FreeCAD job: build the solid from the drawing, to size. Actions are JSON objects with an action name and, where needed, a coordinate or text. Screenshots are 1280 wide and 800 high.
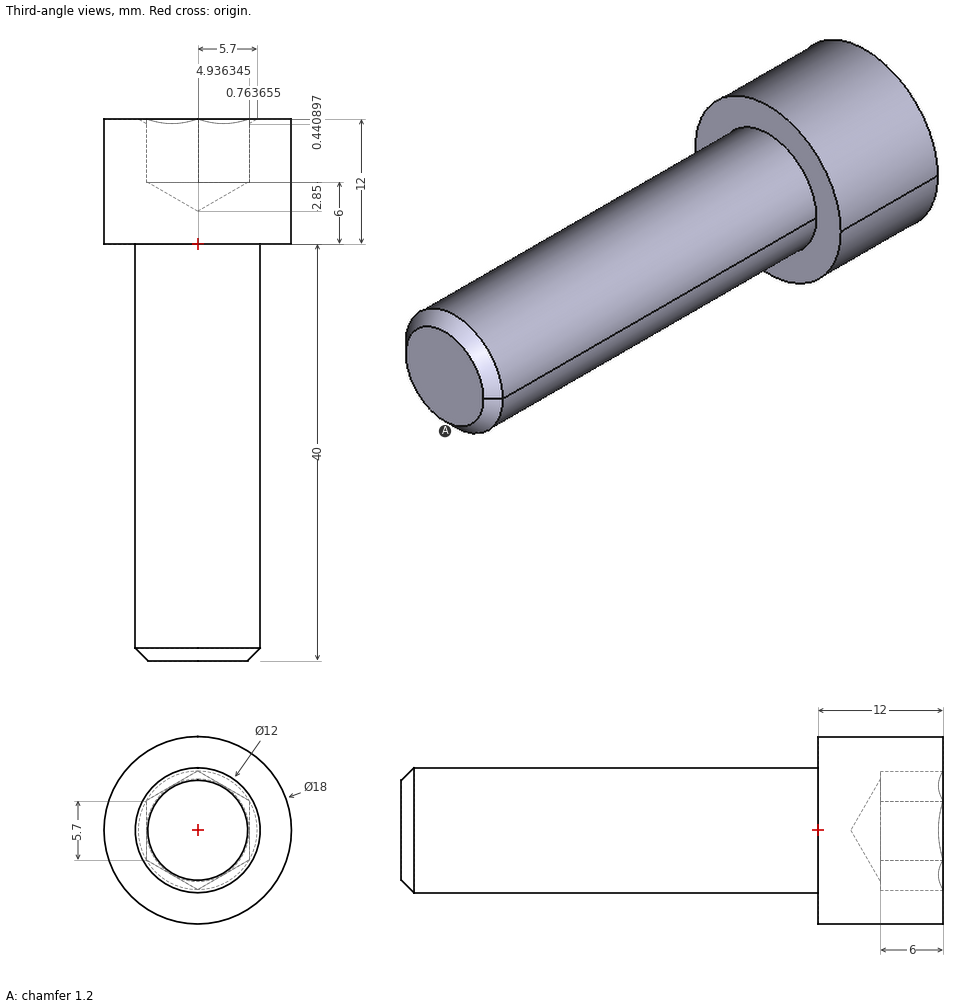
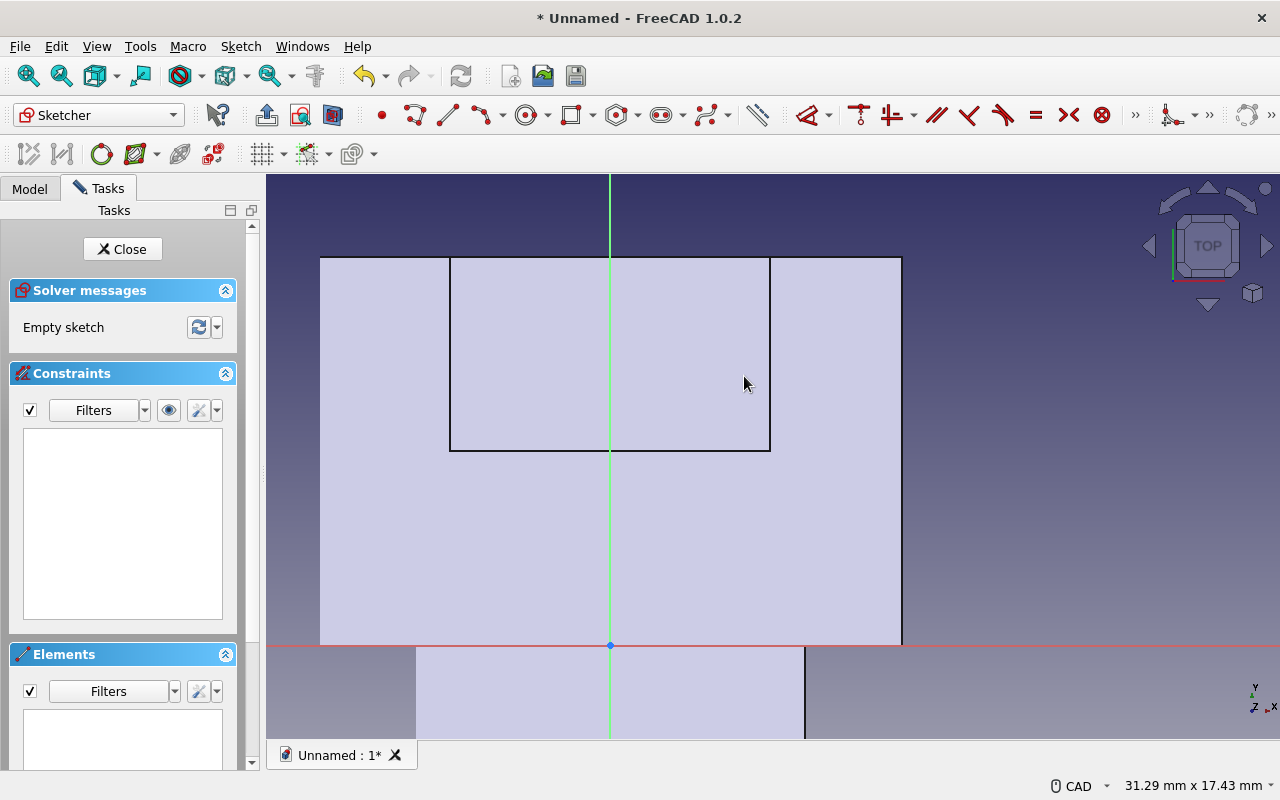
{"action": "left_click", "coordinate": [415, 116]}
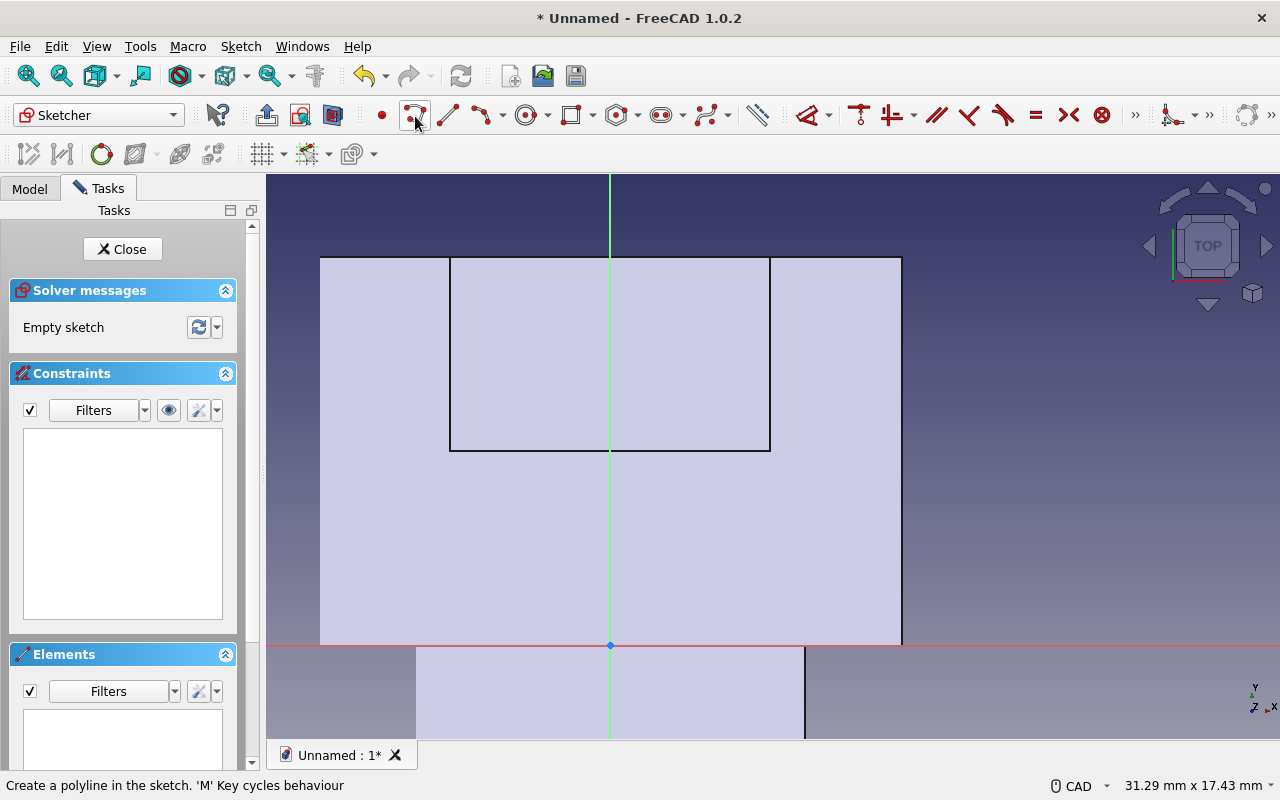
{"action": "left_click", "coordinate": [610, 544]}
{"action": "left_click", "coordinate": [770, 451]}
{"action": "left_click", "coordinate": [619, 451]}
{"action": "left_click", "coordinate": [610, 545]}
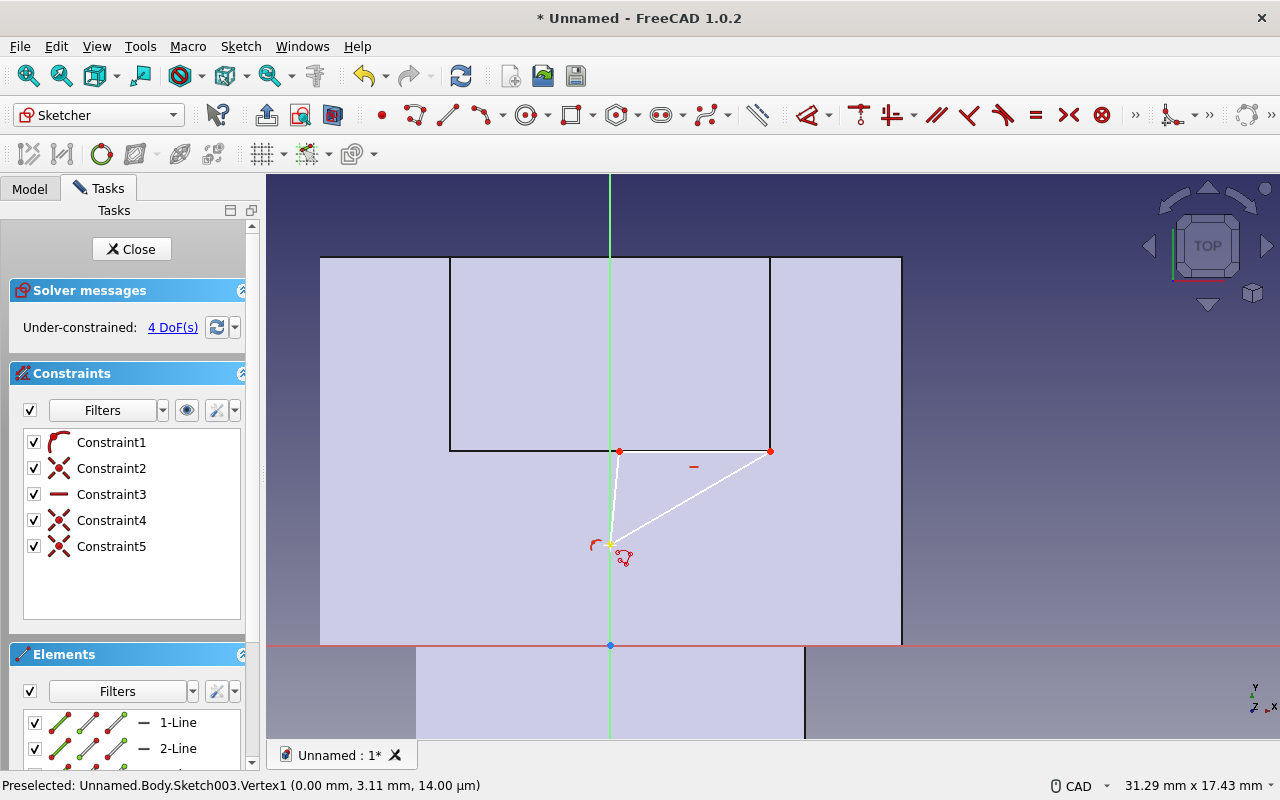
{"action": "left_click", "coordinate": [770, 271]}
{"action": "left_click", "coordinate": [795, 257]}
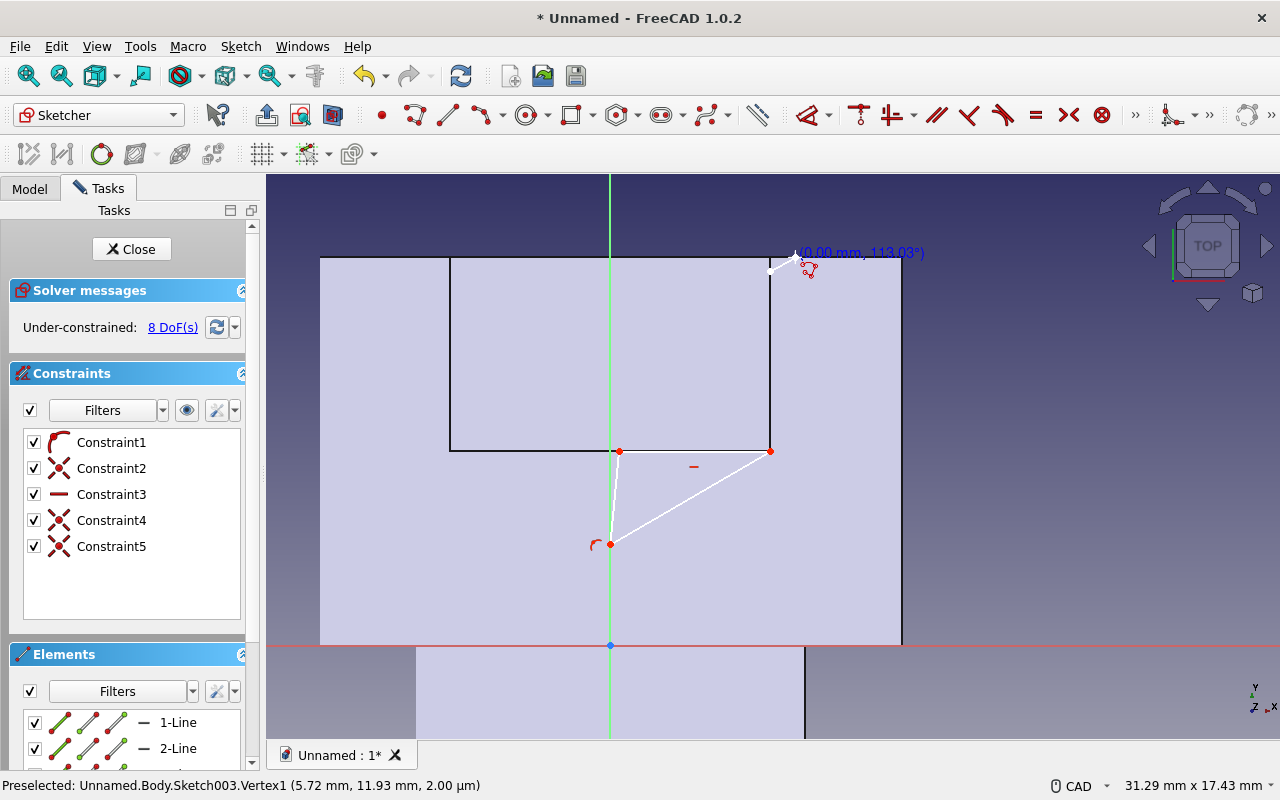
{"action": "scroll", "coordinate": [770, 257], "scroll_direction": "up", "scroll_amount": 2}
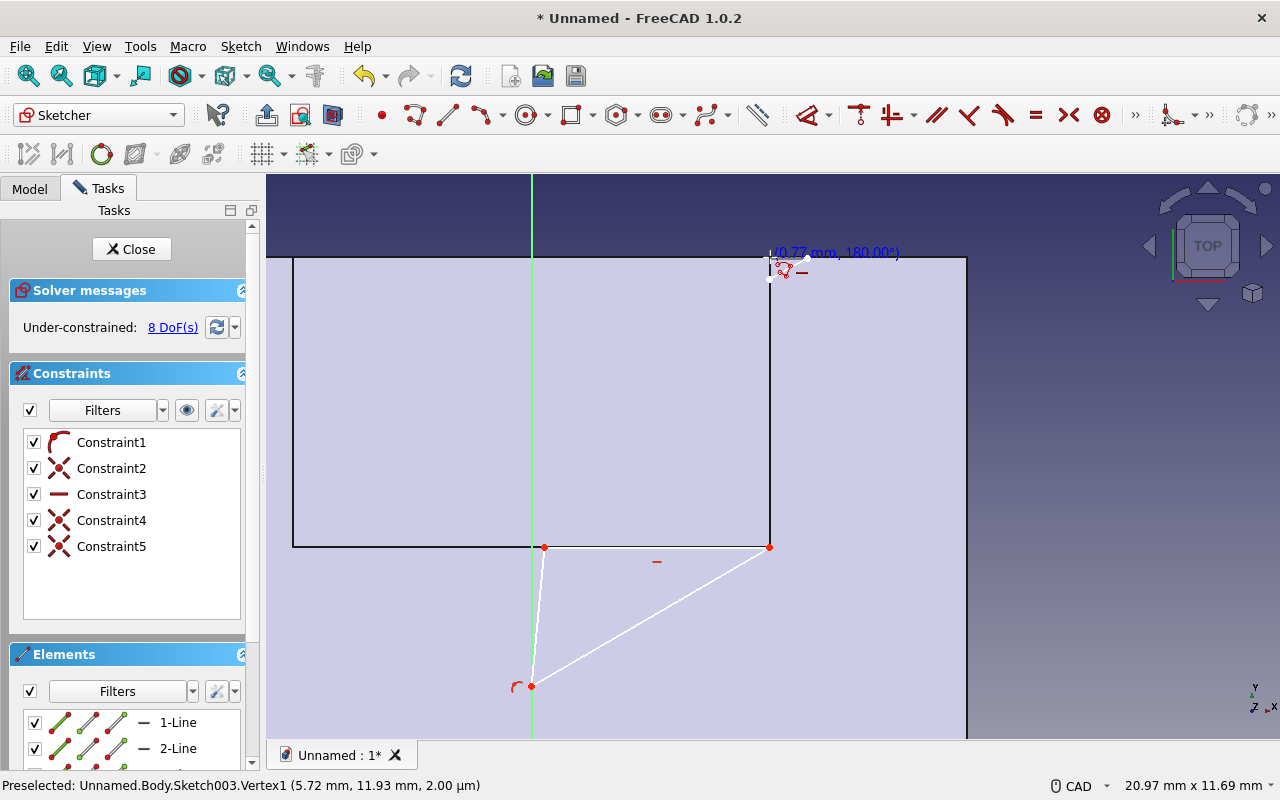
{"action": "left_click", "coordinate": [770, 257]}
{"action": "left_click", "coordinate": [770, 279]}
{"action": "key", "text": "Escape"}
{"action": "key", "text": "Escape"}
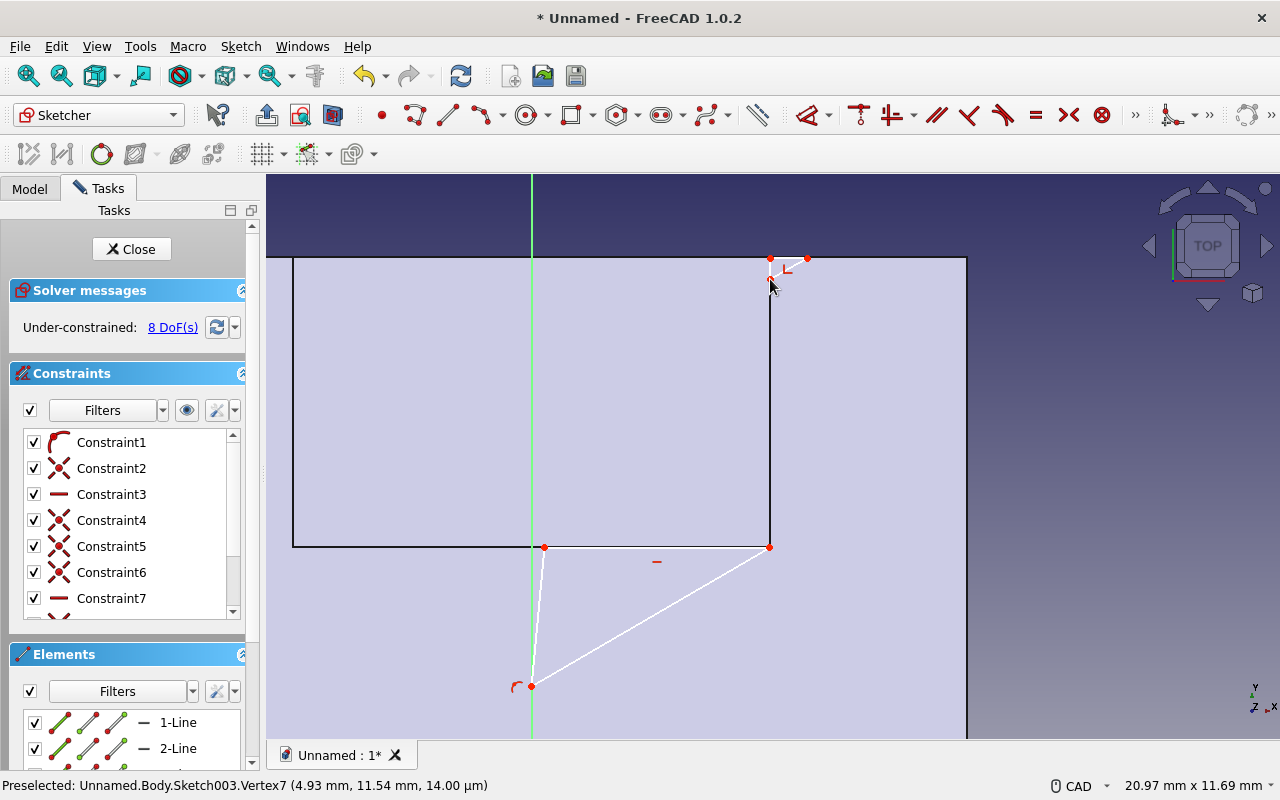
{"action": "scroll", "coordinate": [541, 589], "scroll_direction": "up", "scroll_amount": 3}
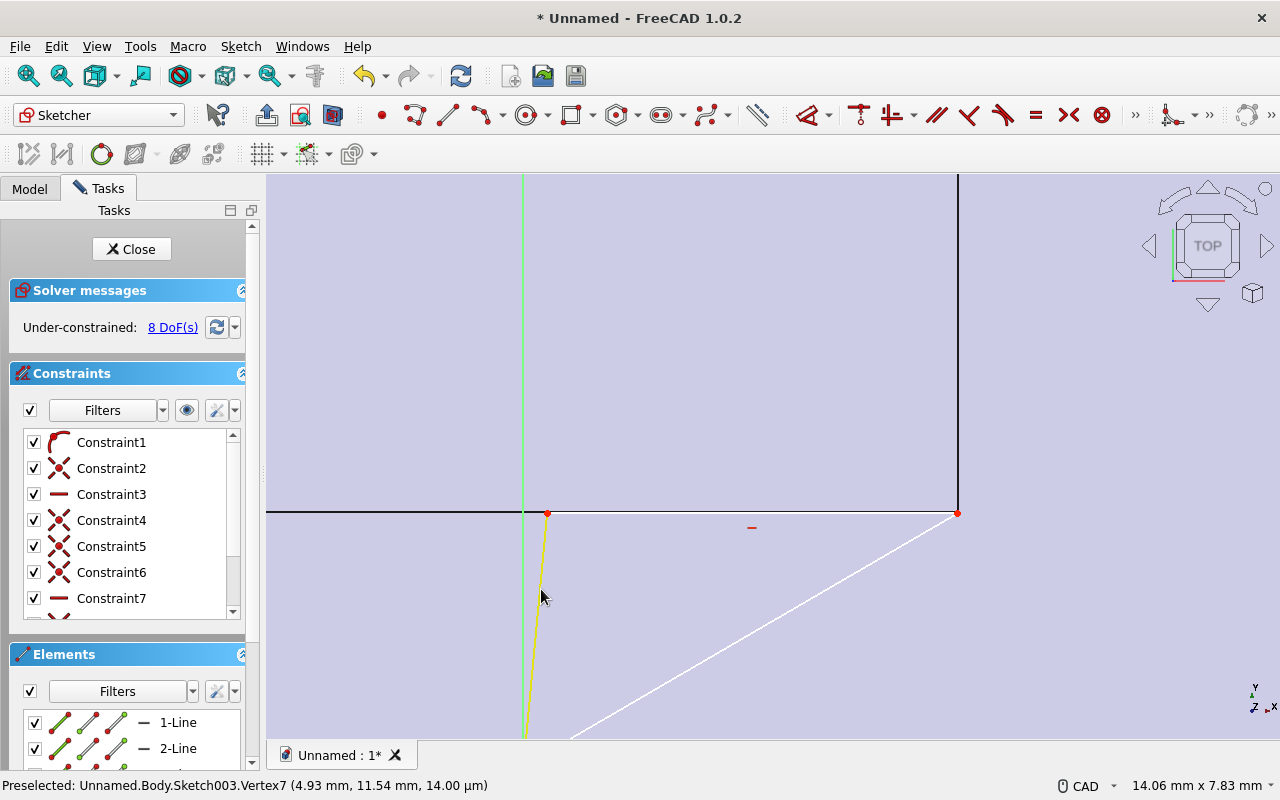
{"action": "left_click", "coordinate": [540, 589]}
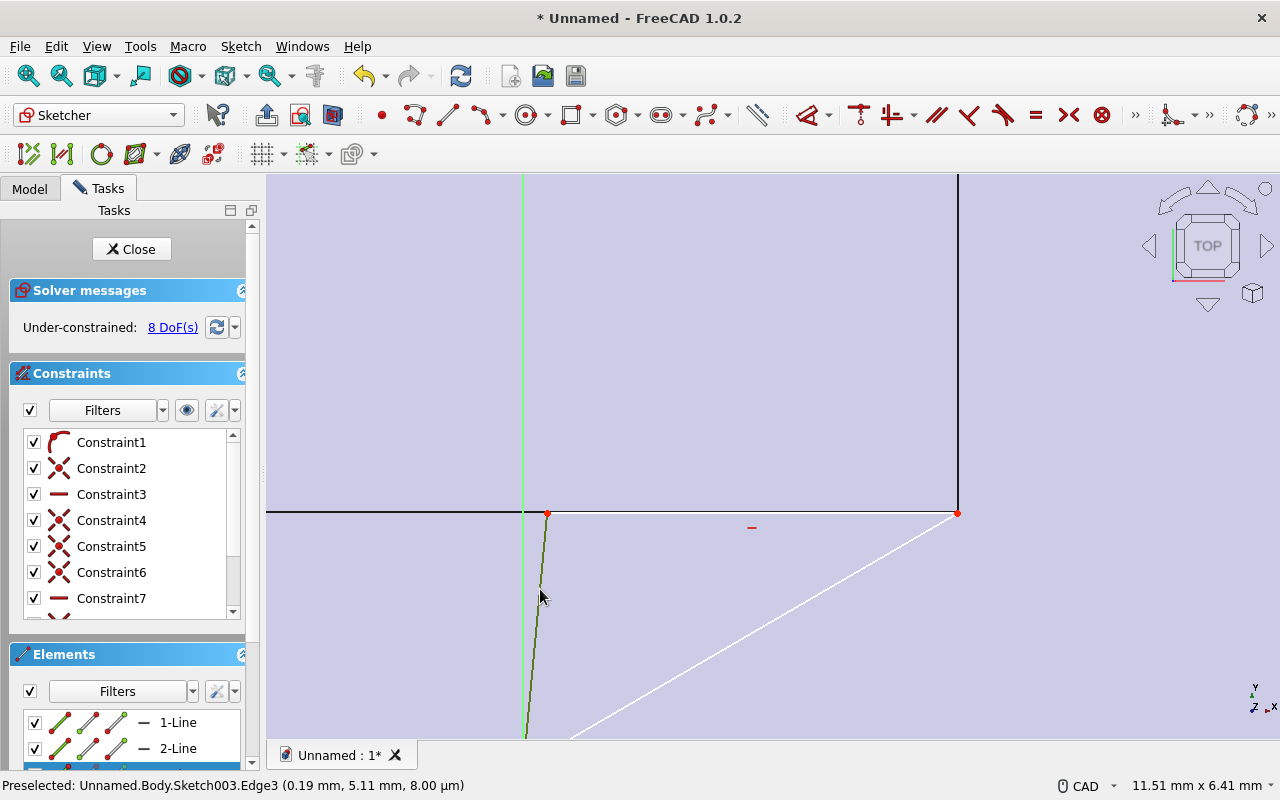
{"action": "key", "text": "v"}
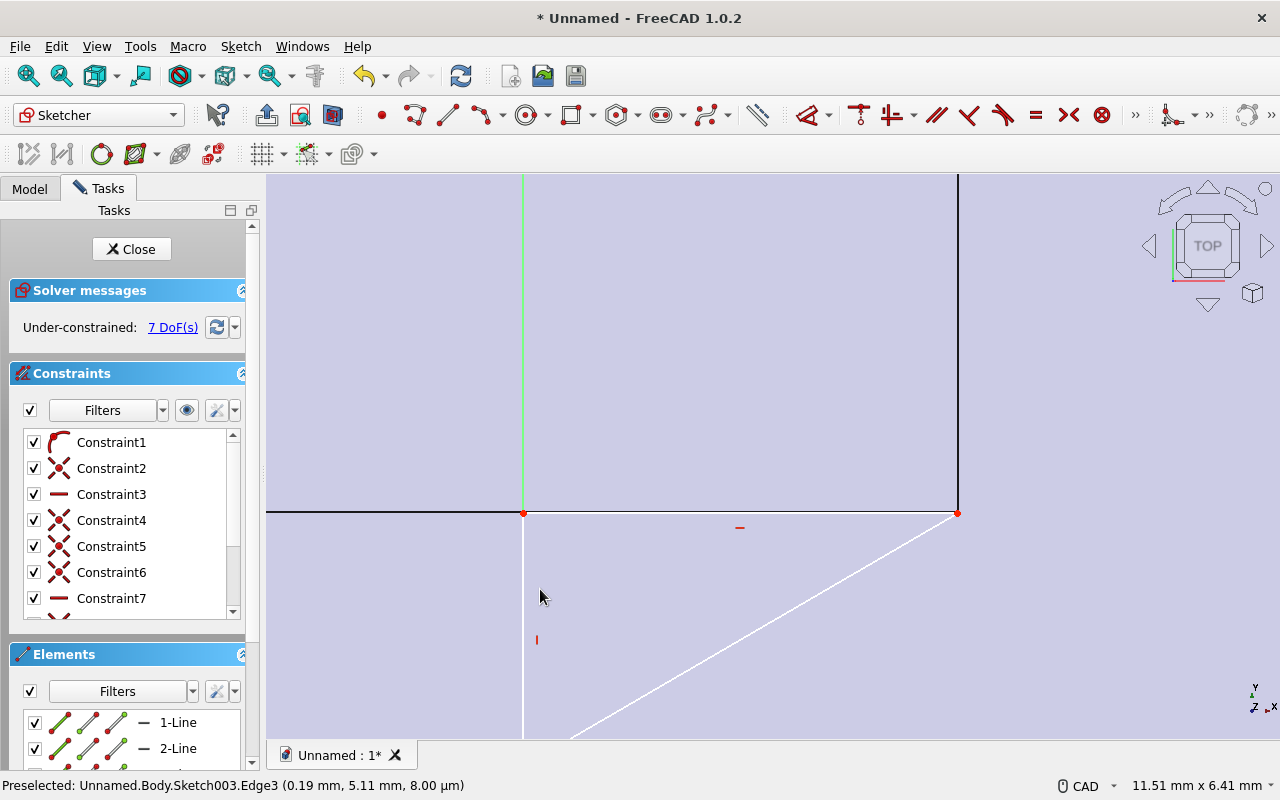
{"action": "left_click", "coordinate": [806, 116]}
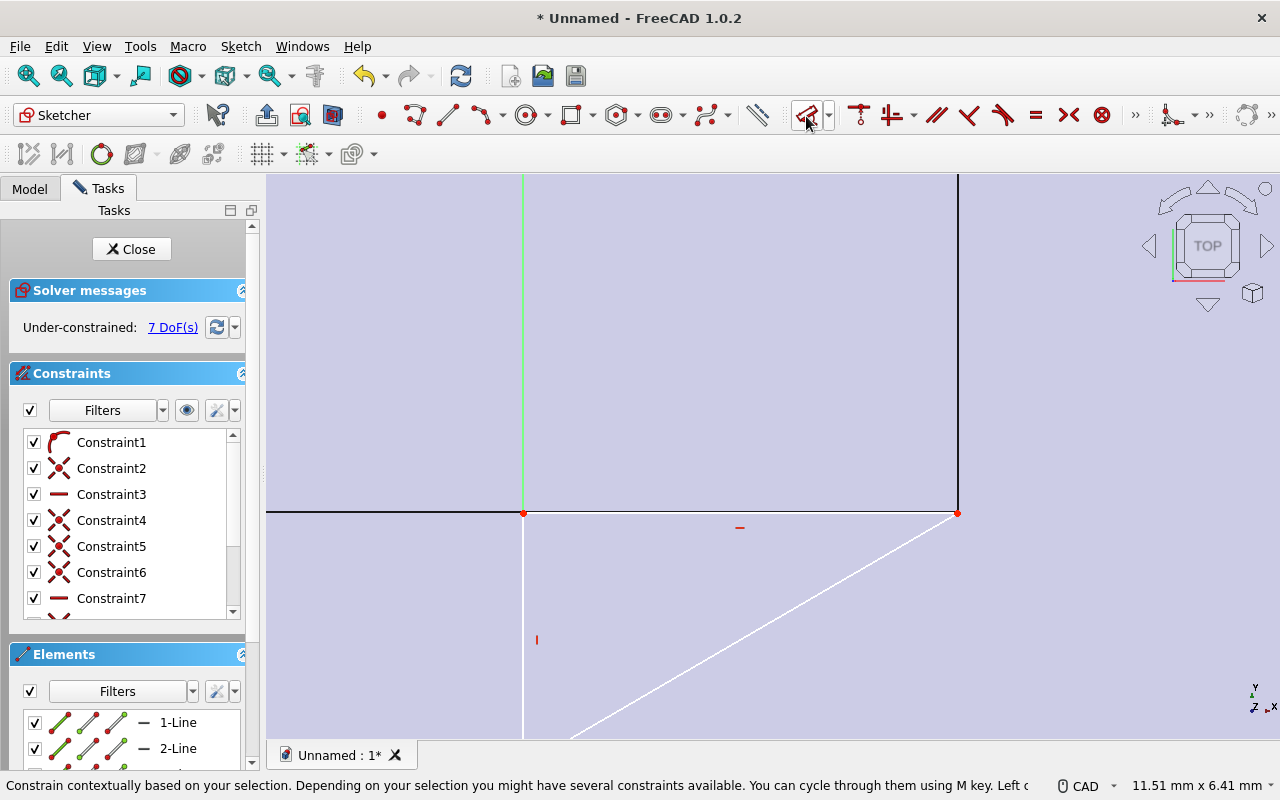
{"action": "left_click", "coordinate": [958, 513]}
{"action": "left_click", "coordinate": [489, 612]}